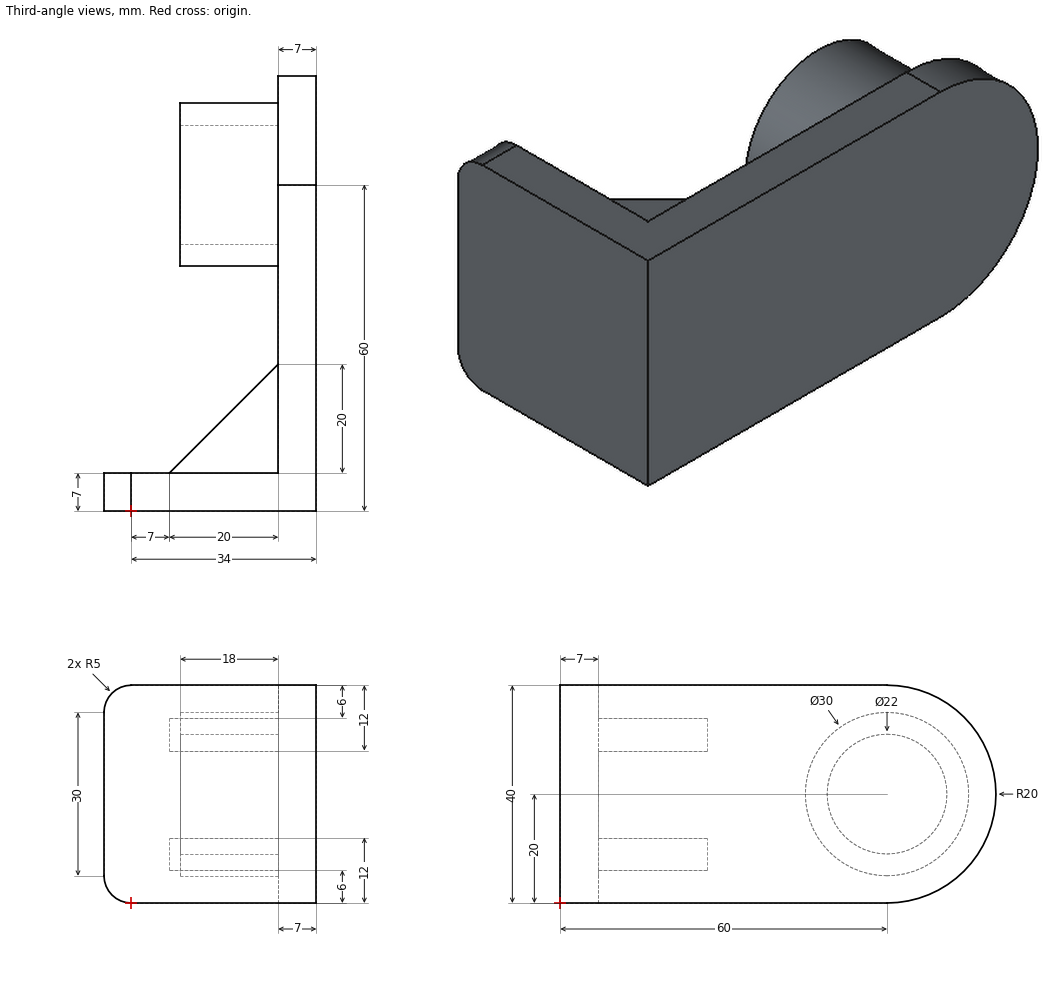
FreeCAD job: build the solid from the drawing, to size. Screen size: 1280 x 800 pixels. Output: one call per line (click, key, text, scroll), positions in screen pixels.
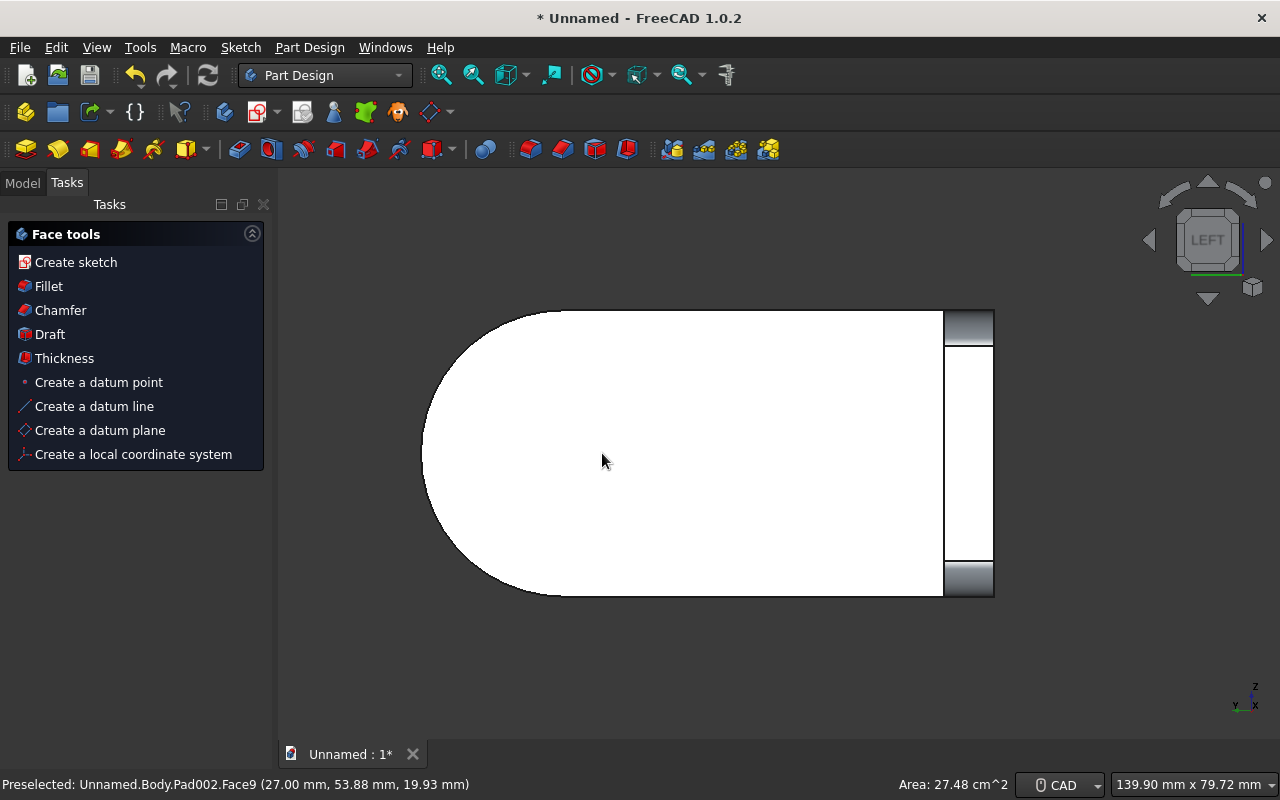
click(258, 112)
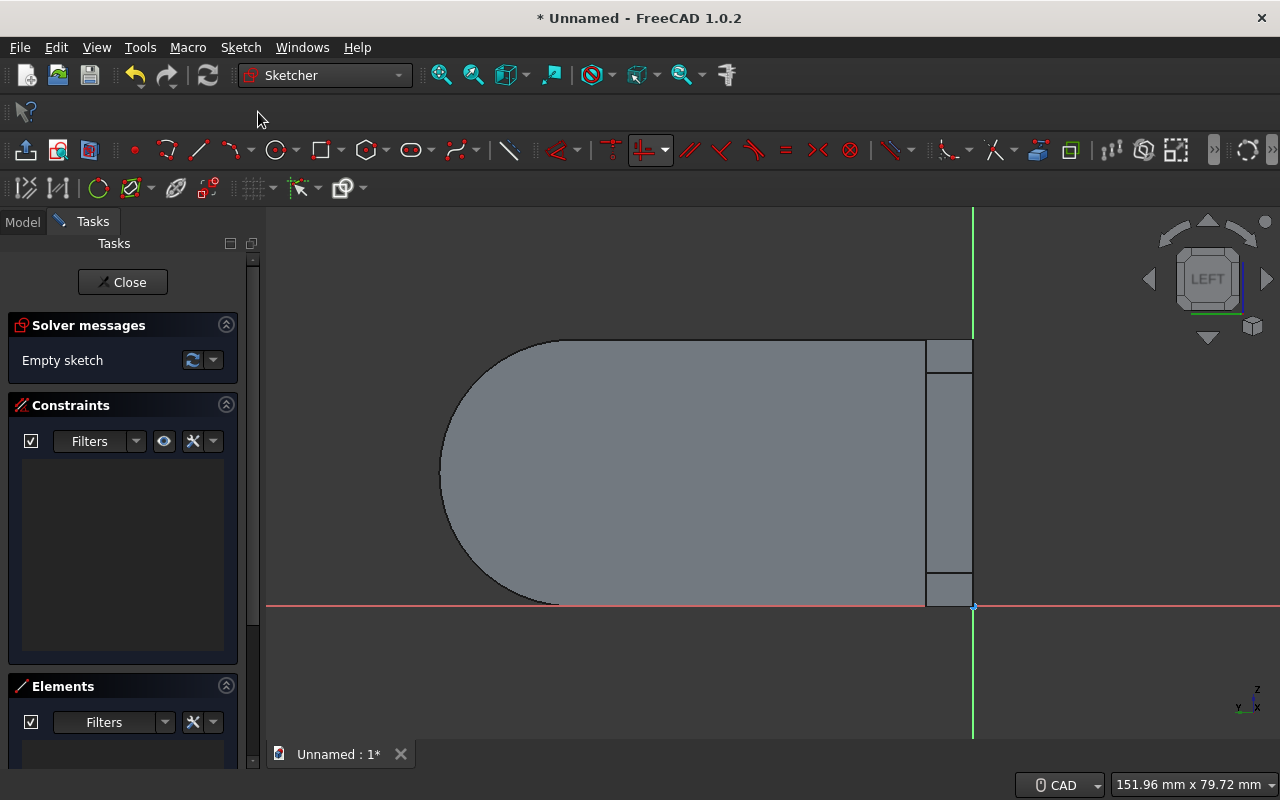
scroll(413, 473, up, 3)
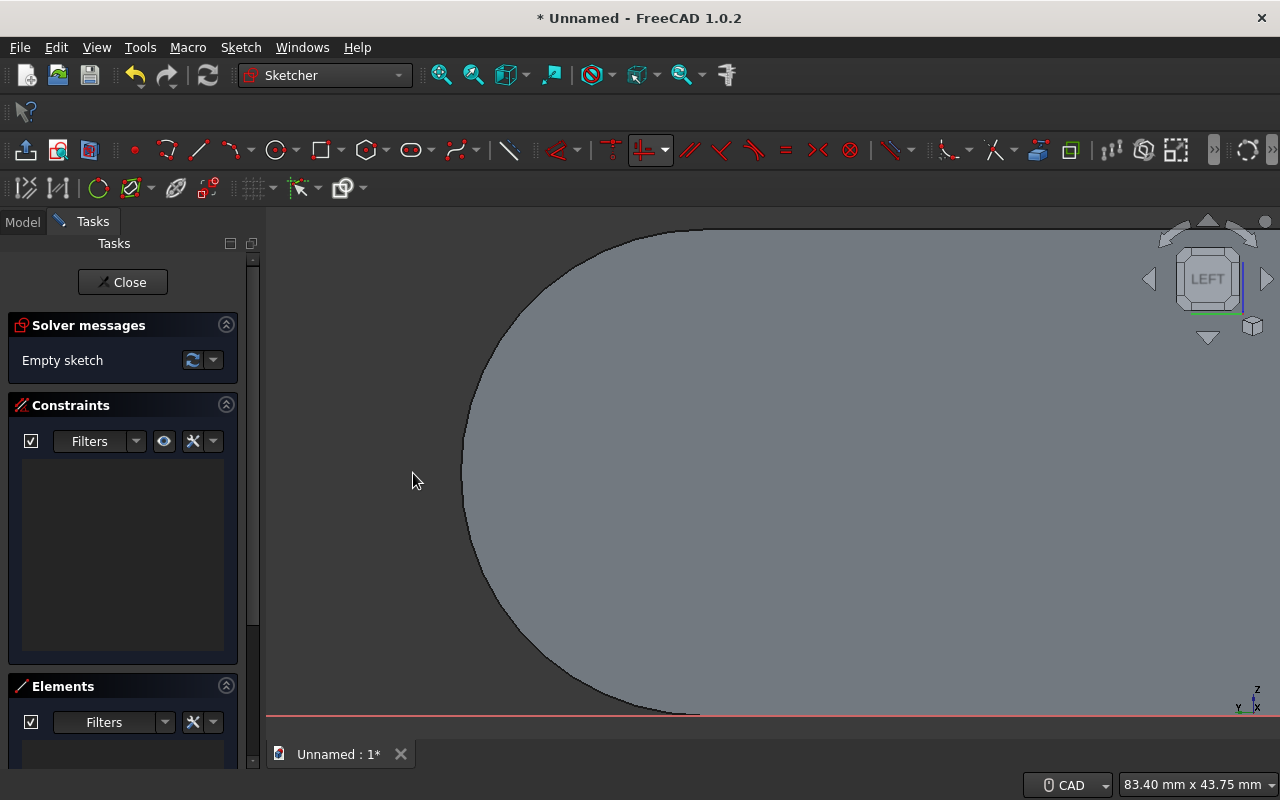
click(276, 150)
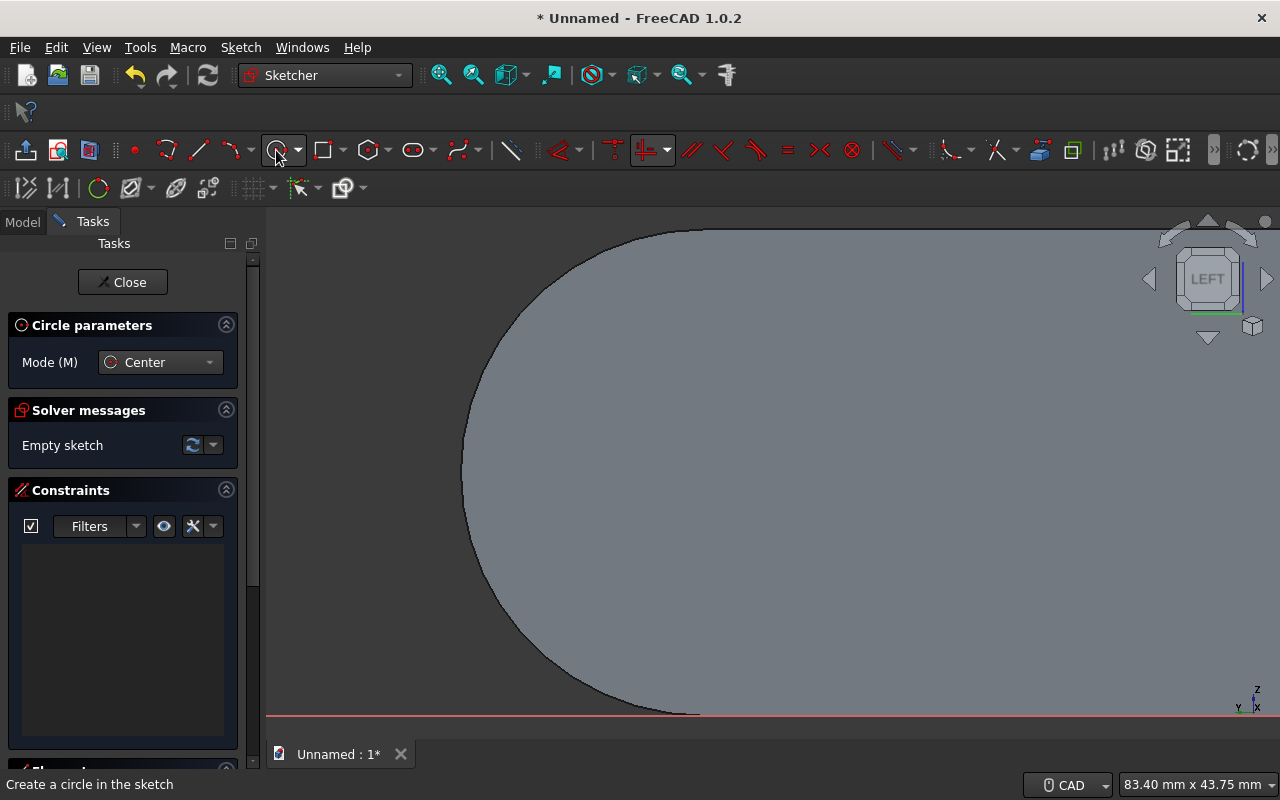
click(704, 473)
click(833, 344)
key(Escape)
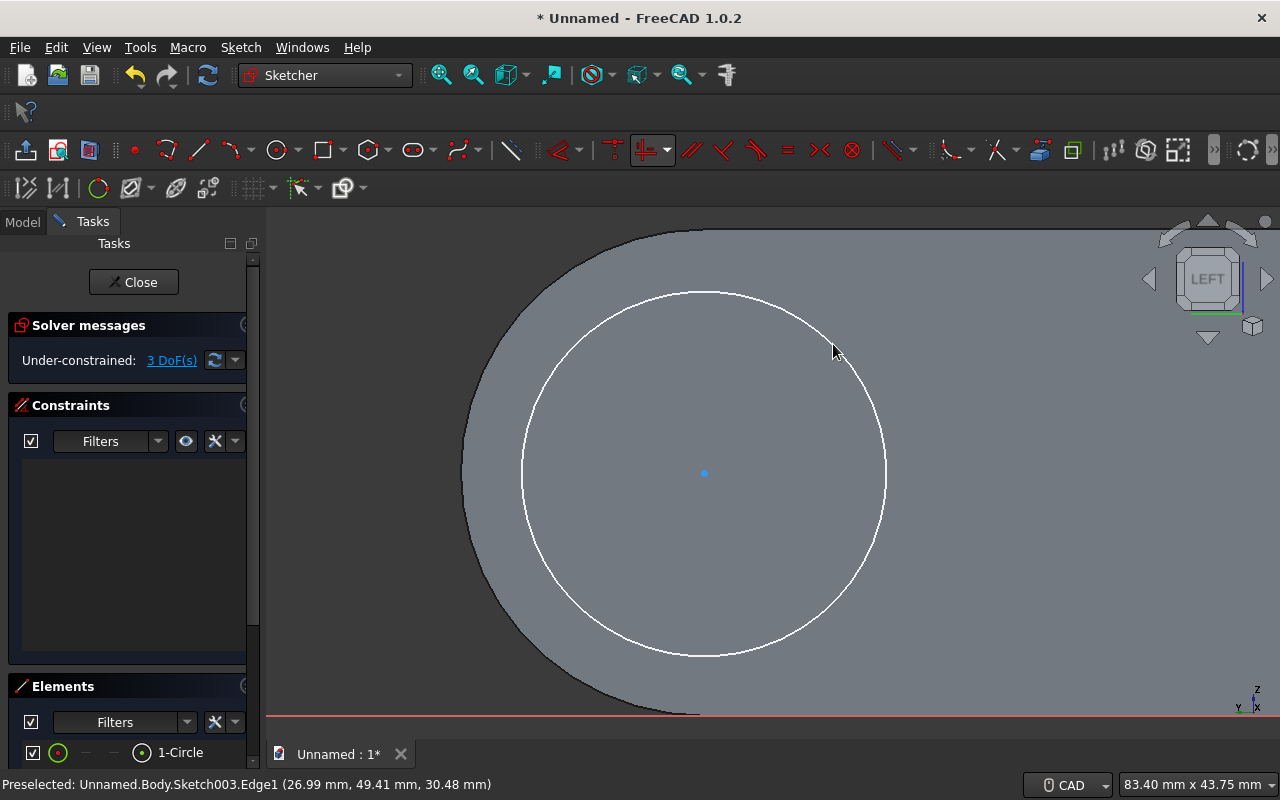
click(558, 150)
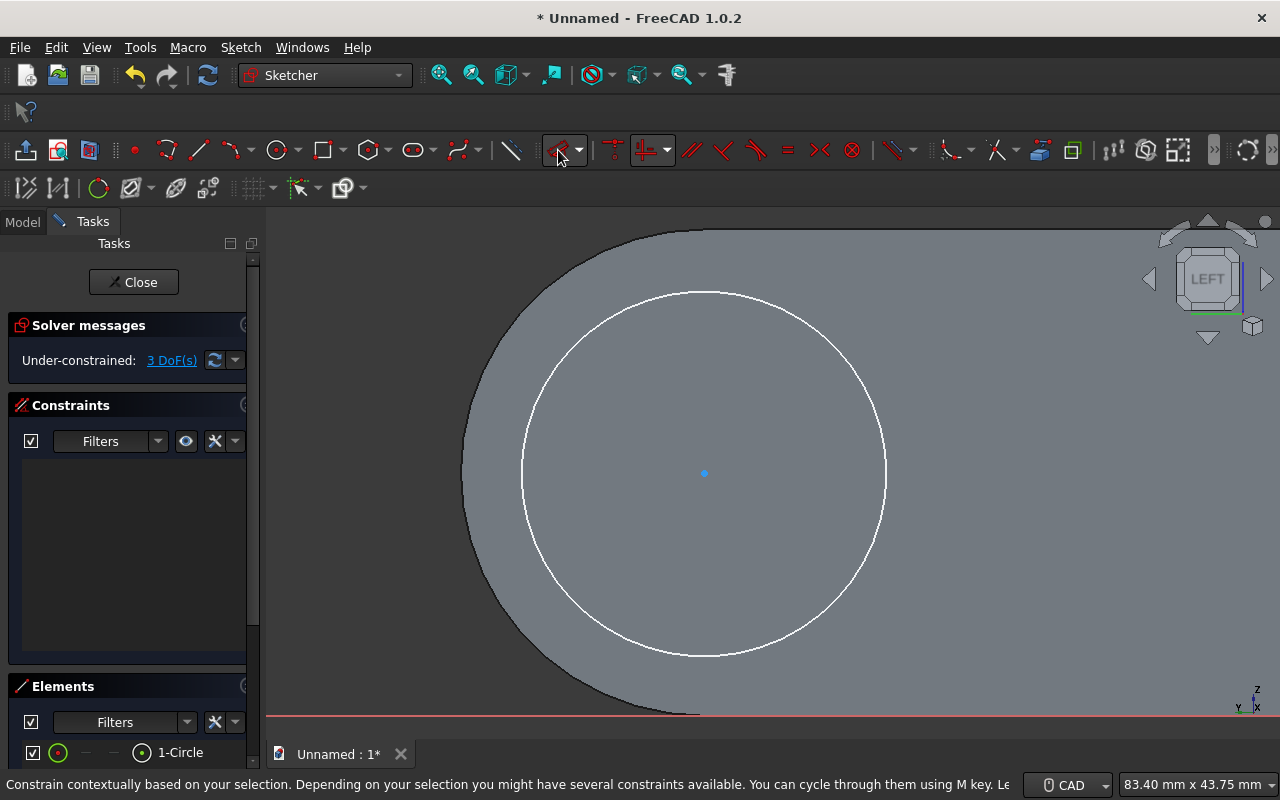
click(833, 345)
click(856, 322)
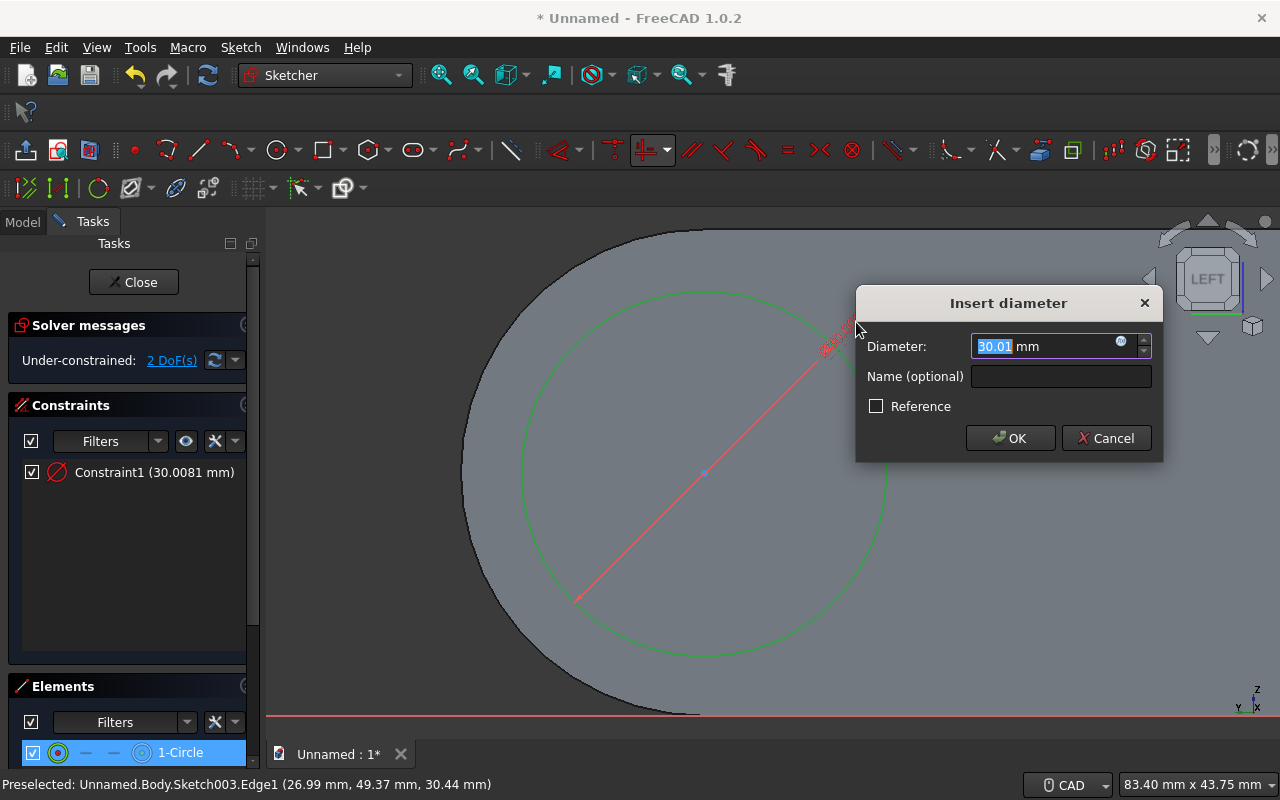
text(30)
key(Return)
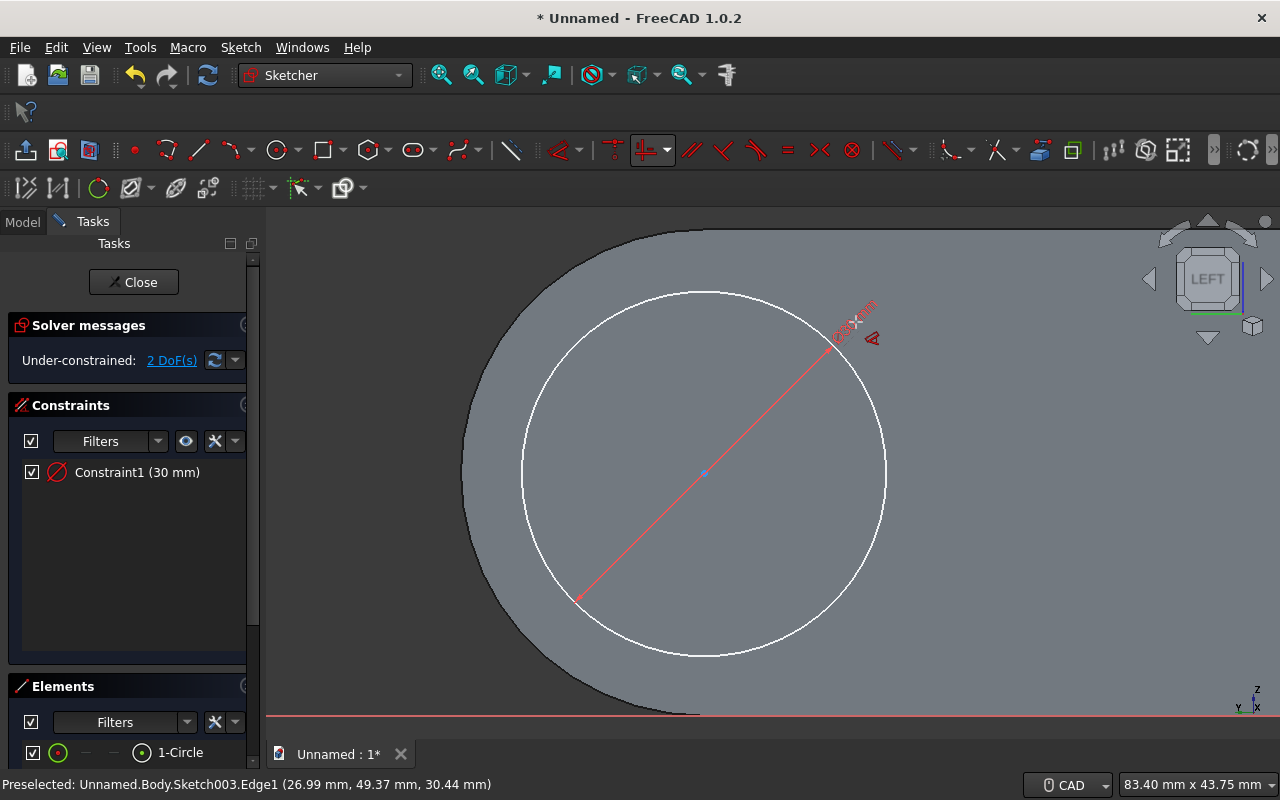
click(704, 474)
click(910, 440)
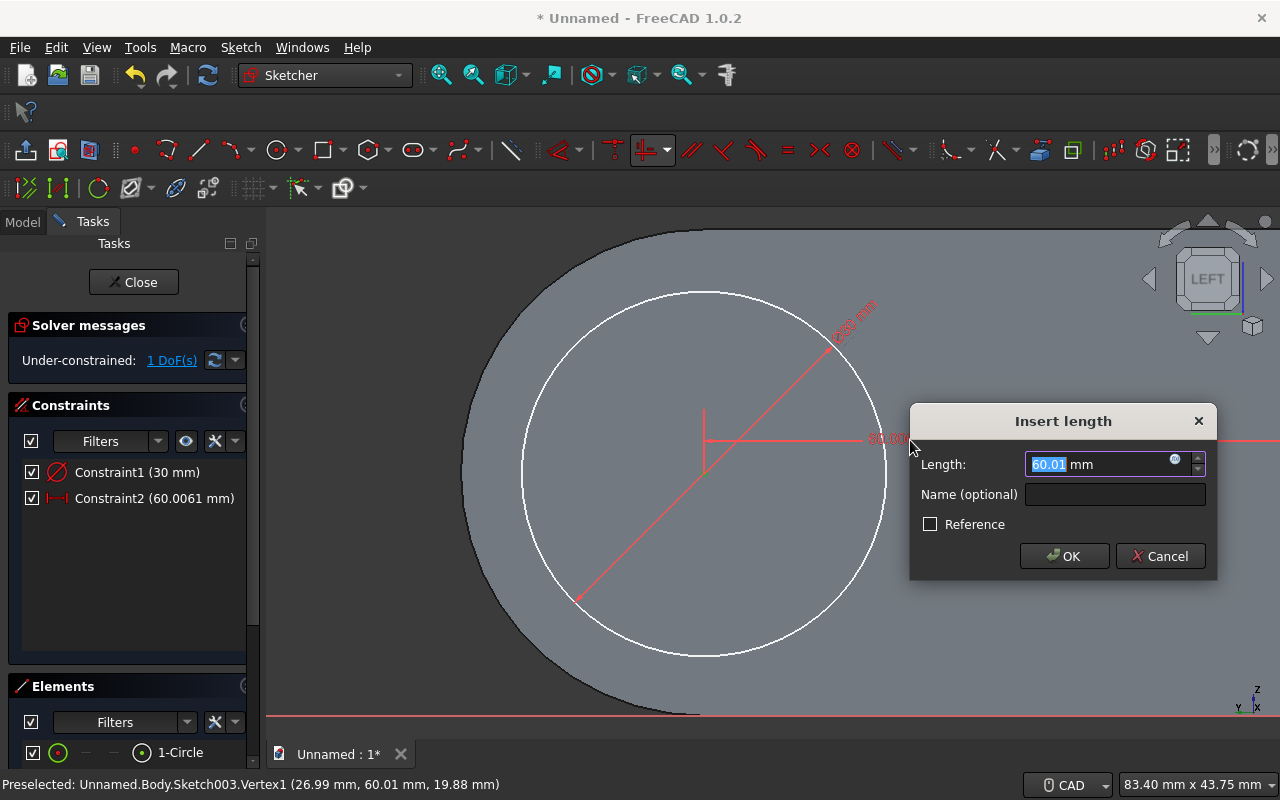
text(60)
key(Return)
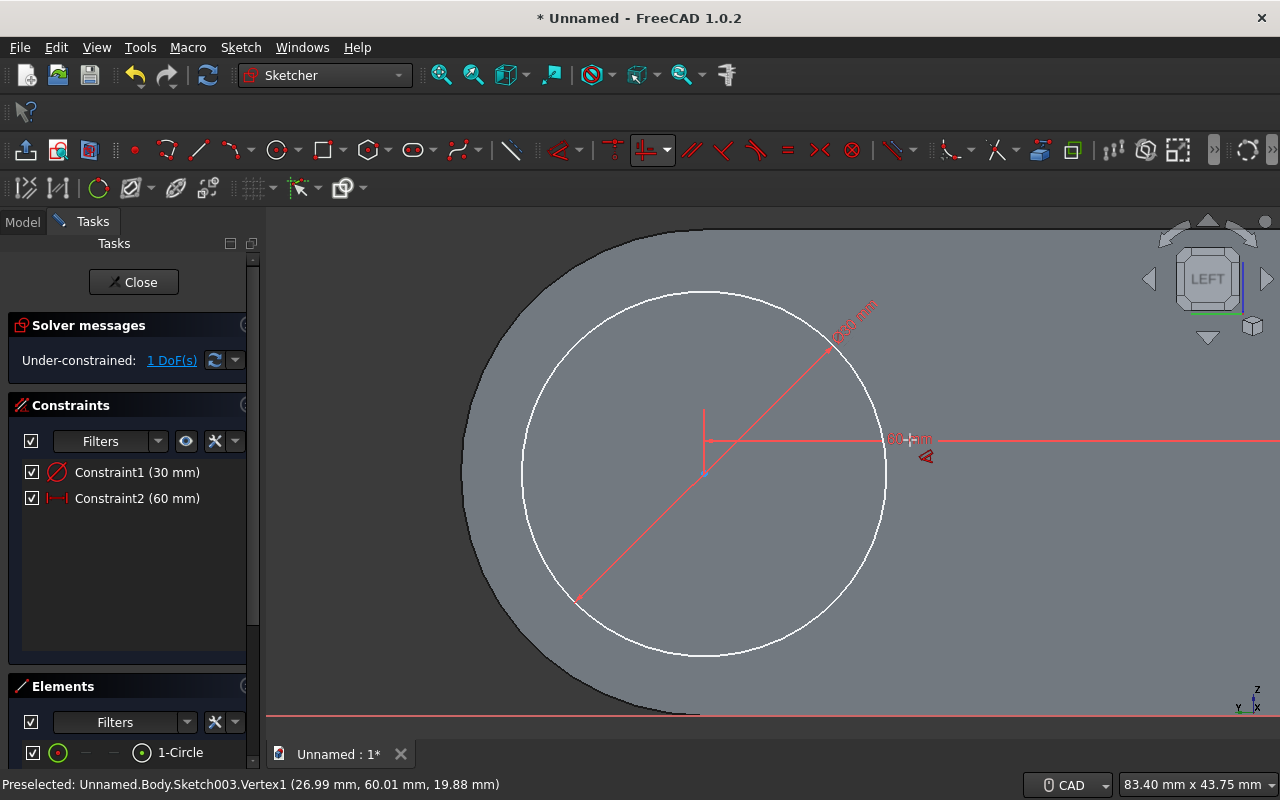
click(704, 474)
click(670, 592)